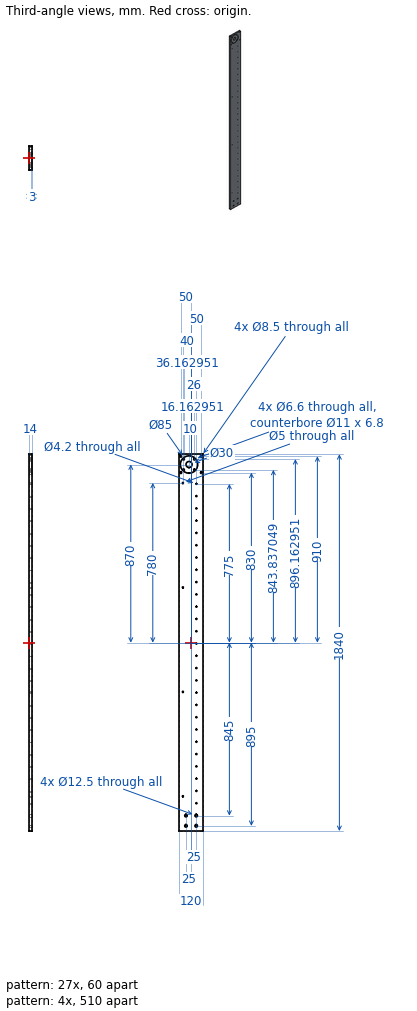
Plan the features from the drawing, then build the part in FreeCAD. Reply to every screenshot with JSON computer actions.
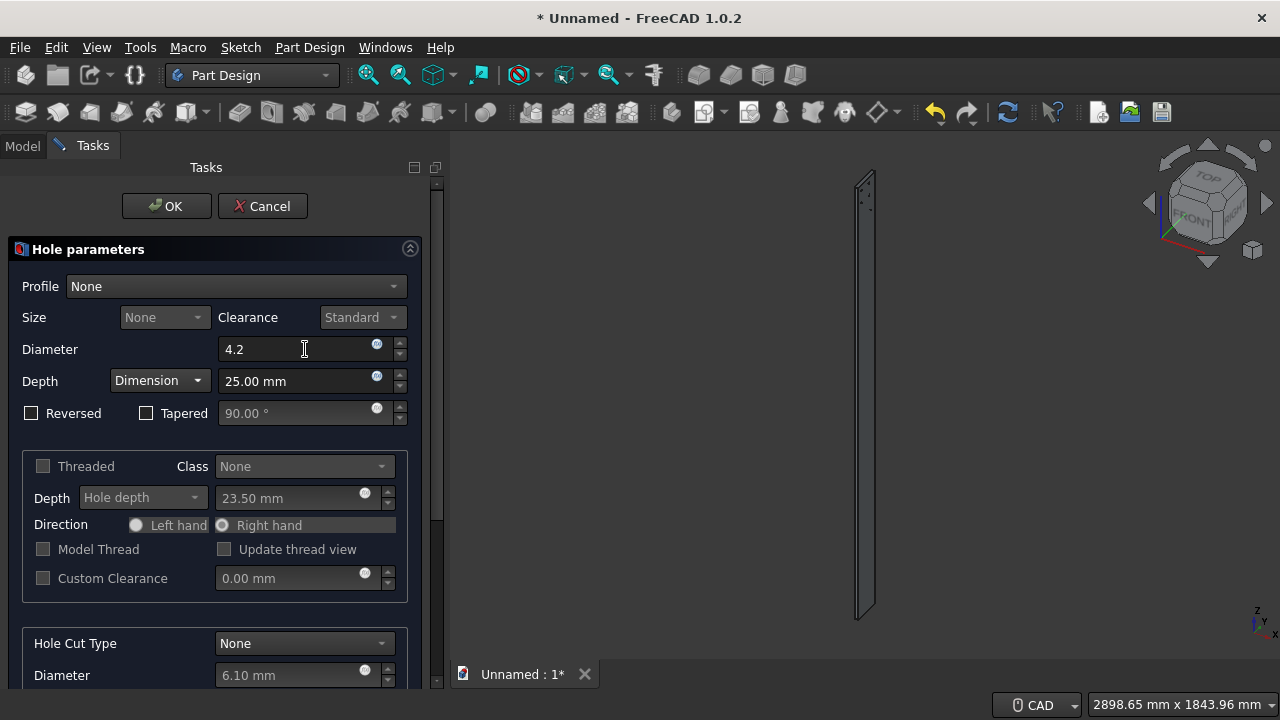
{"action": "left_click", "coordinate": [161, 380]}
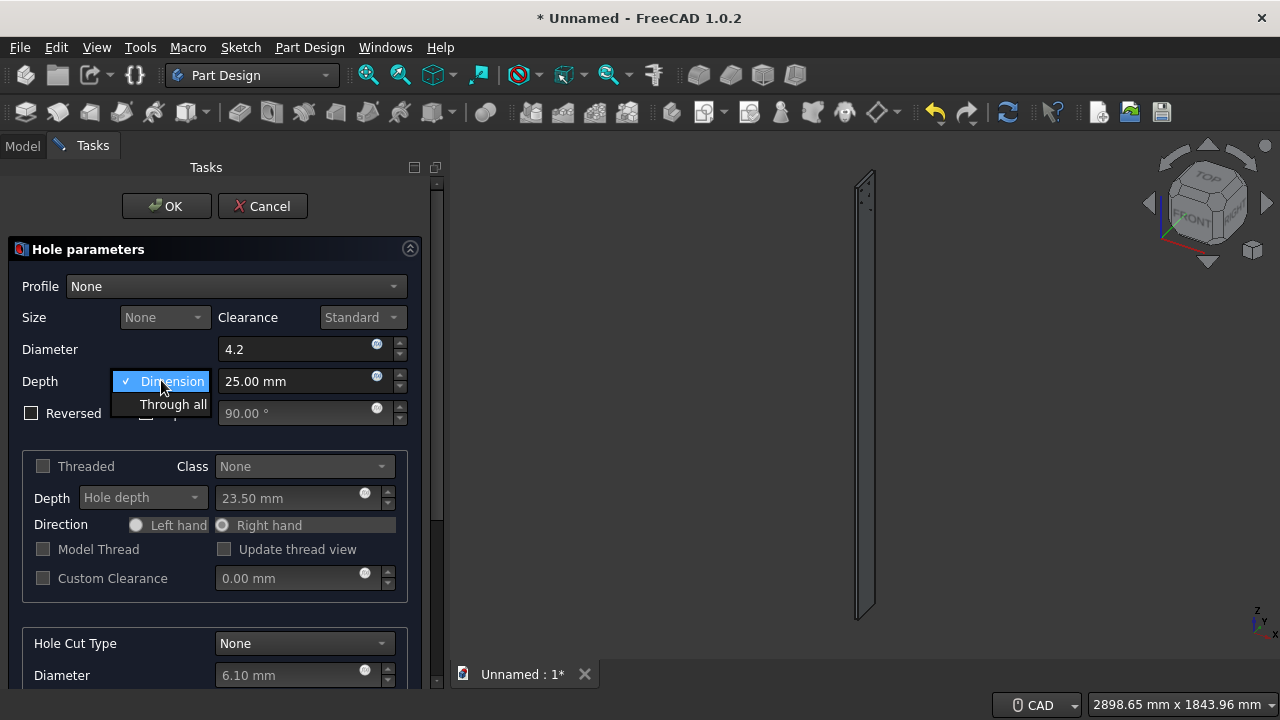
{"action": "left_click", "coordinate": [160, 404]}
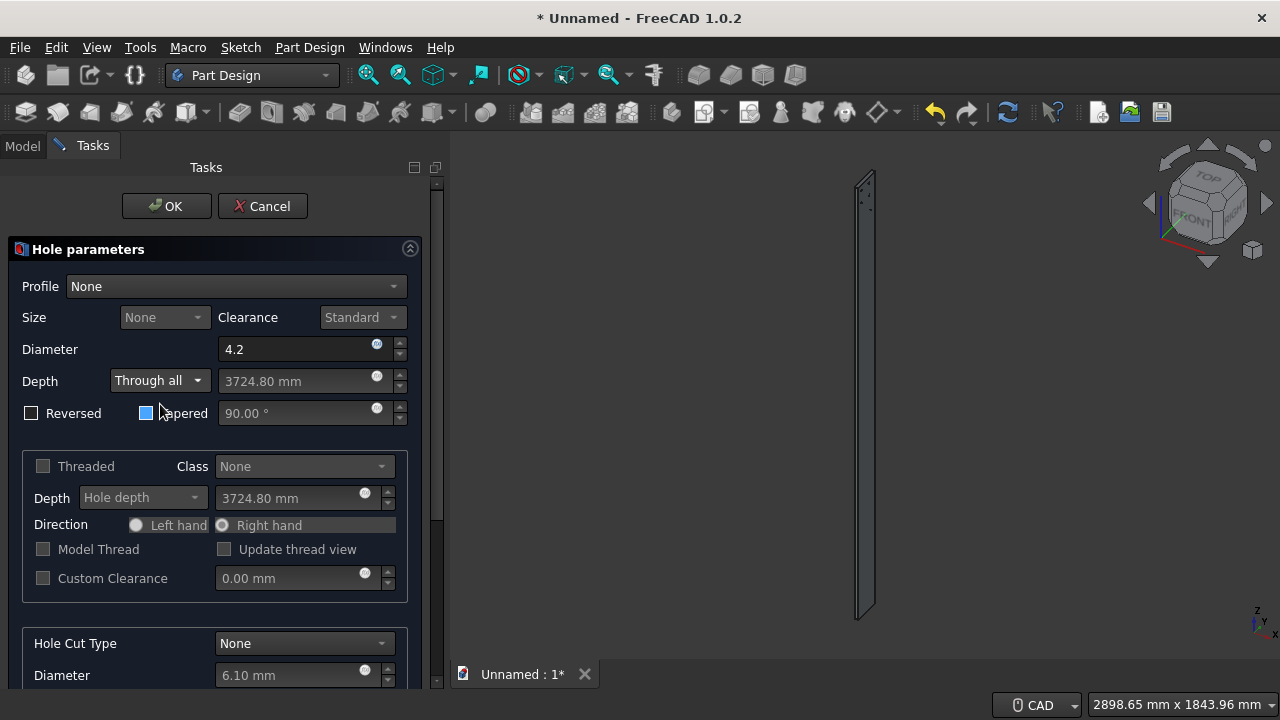
{"action": "left_click", "coordinate": [167, 206]}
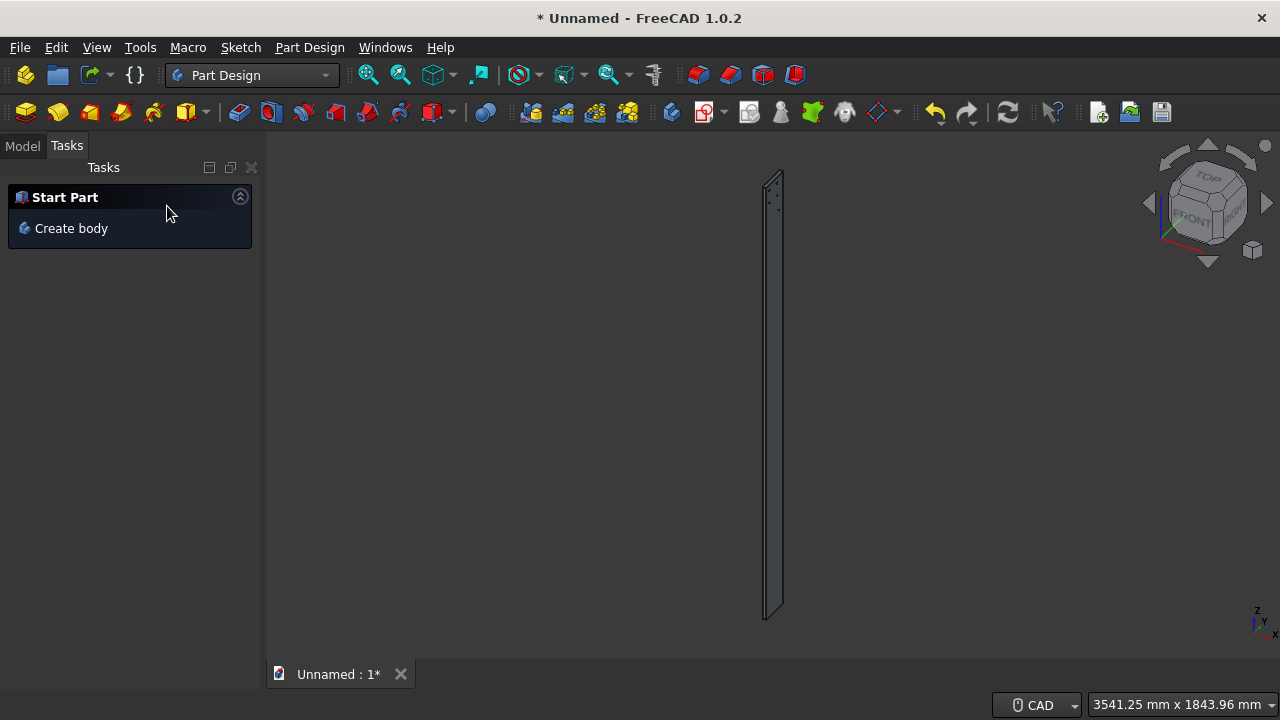
{"action": "left_click", "coordinate": [23, 145]}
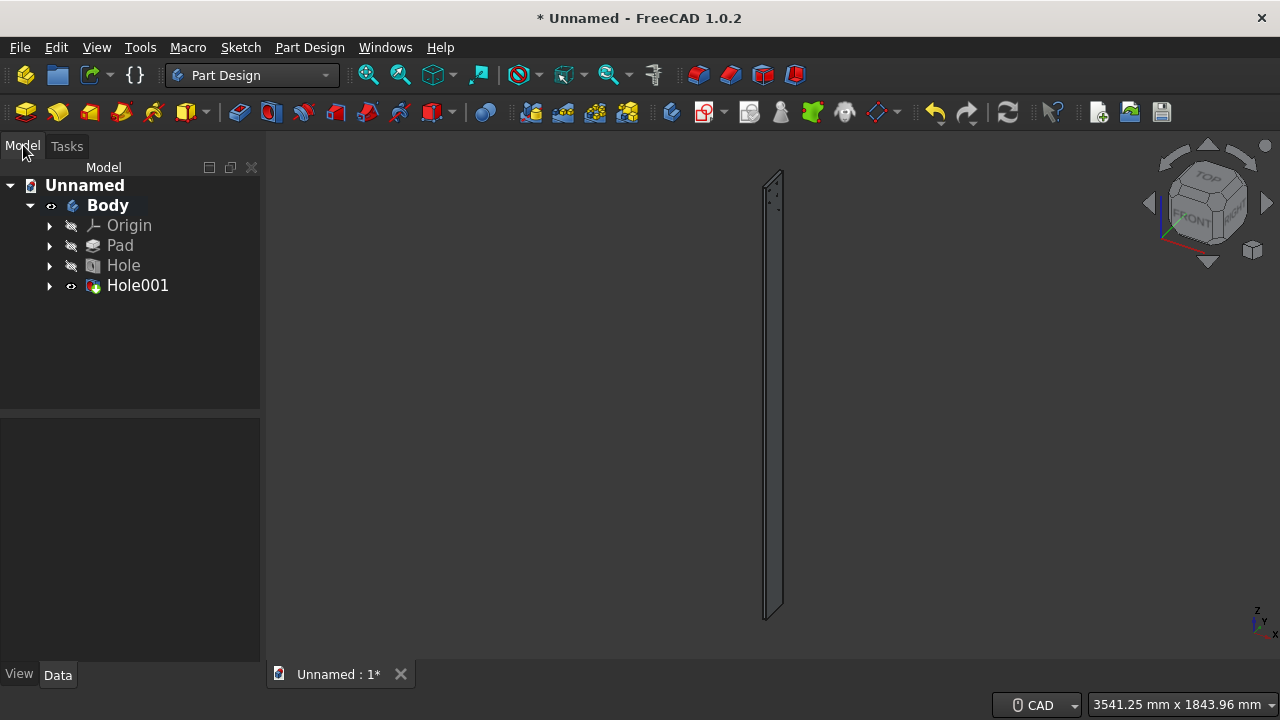
{"action": "left_click", "coordinate": [116, 286]}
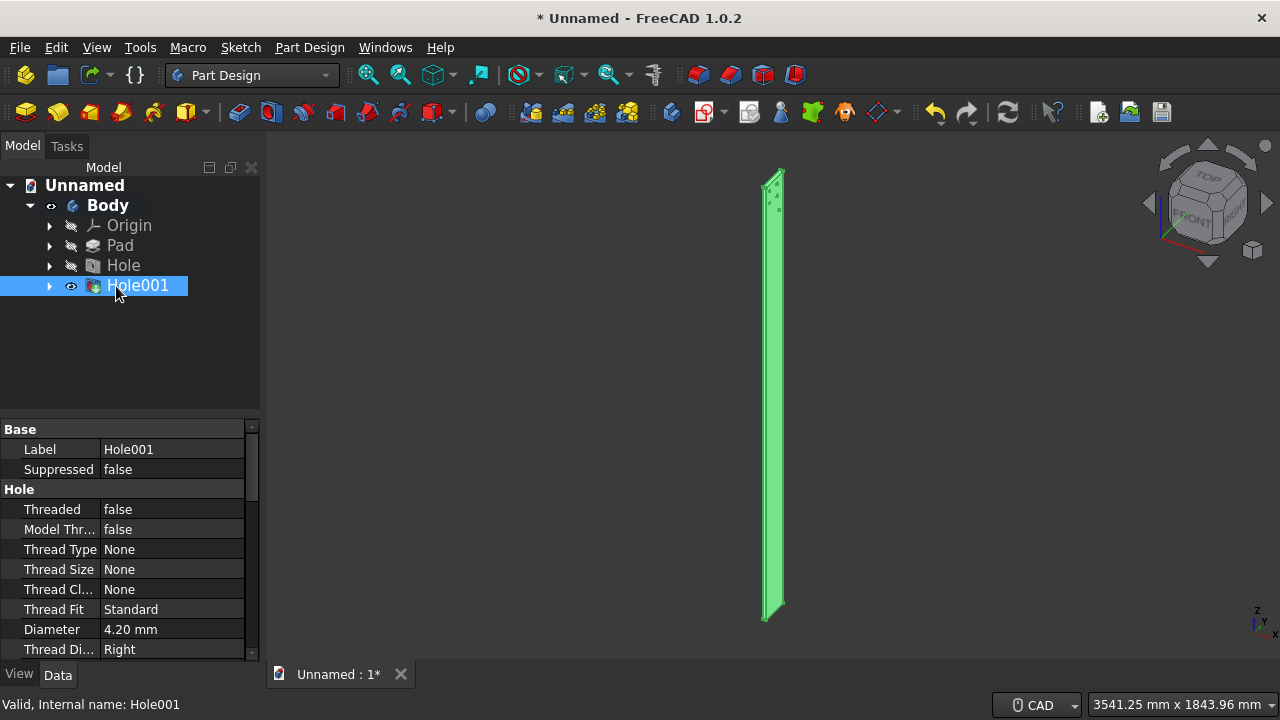
{"action": "left_click", "coordinate": [564, 112]}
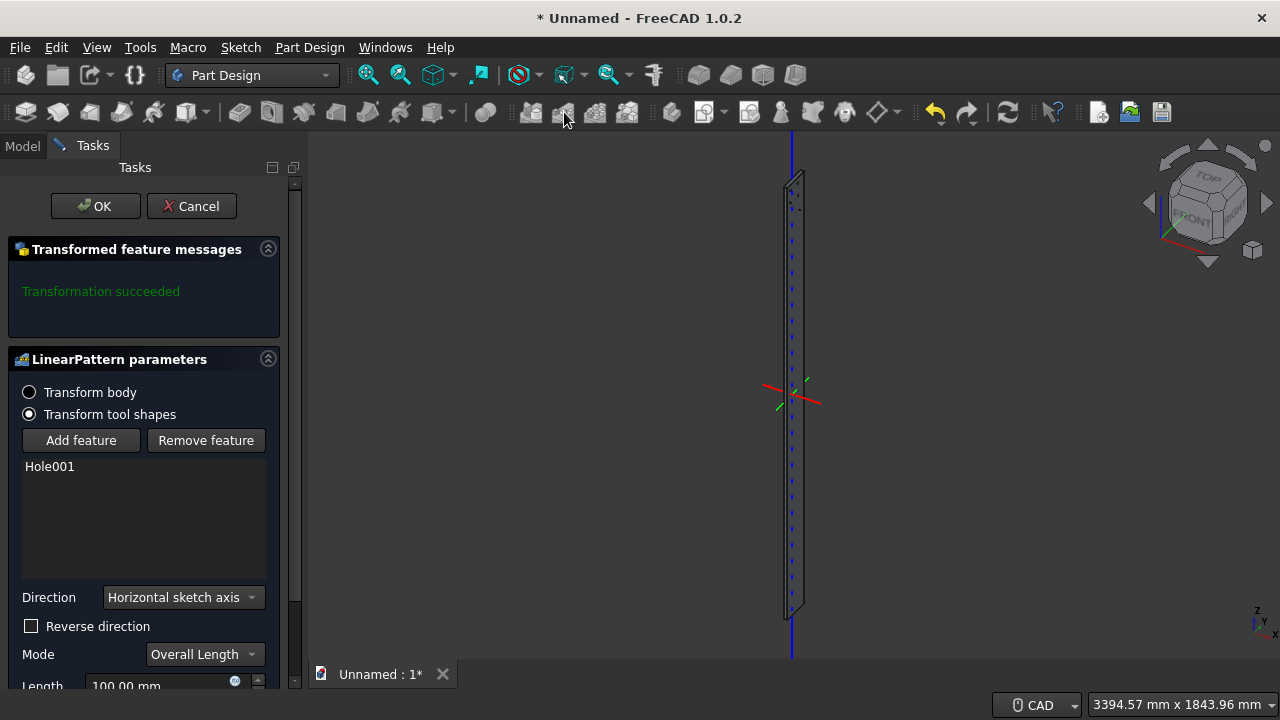
{"action": "left_click", "coordinate": [184, 598]}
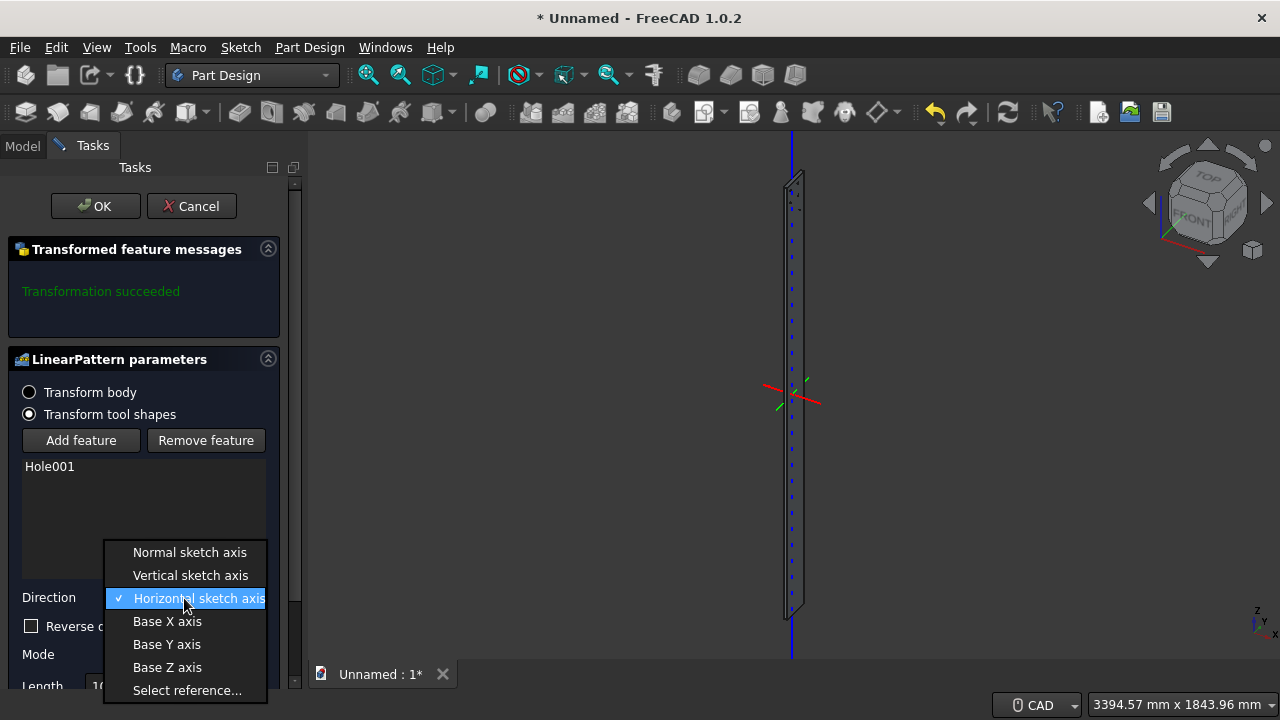
{"action": "left_click", "coordinate": [184, 668]}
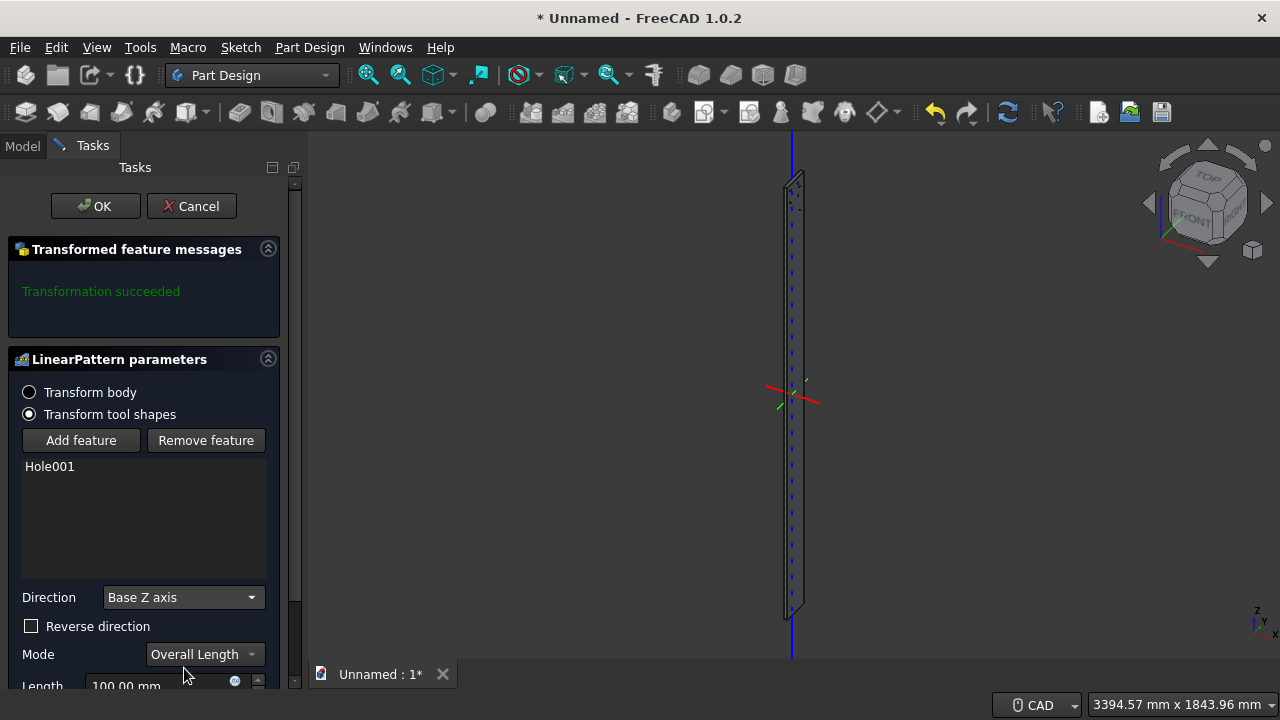
{"action": "left_click", "coordinate": [206, 654]}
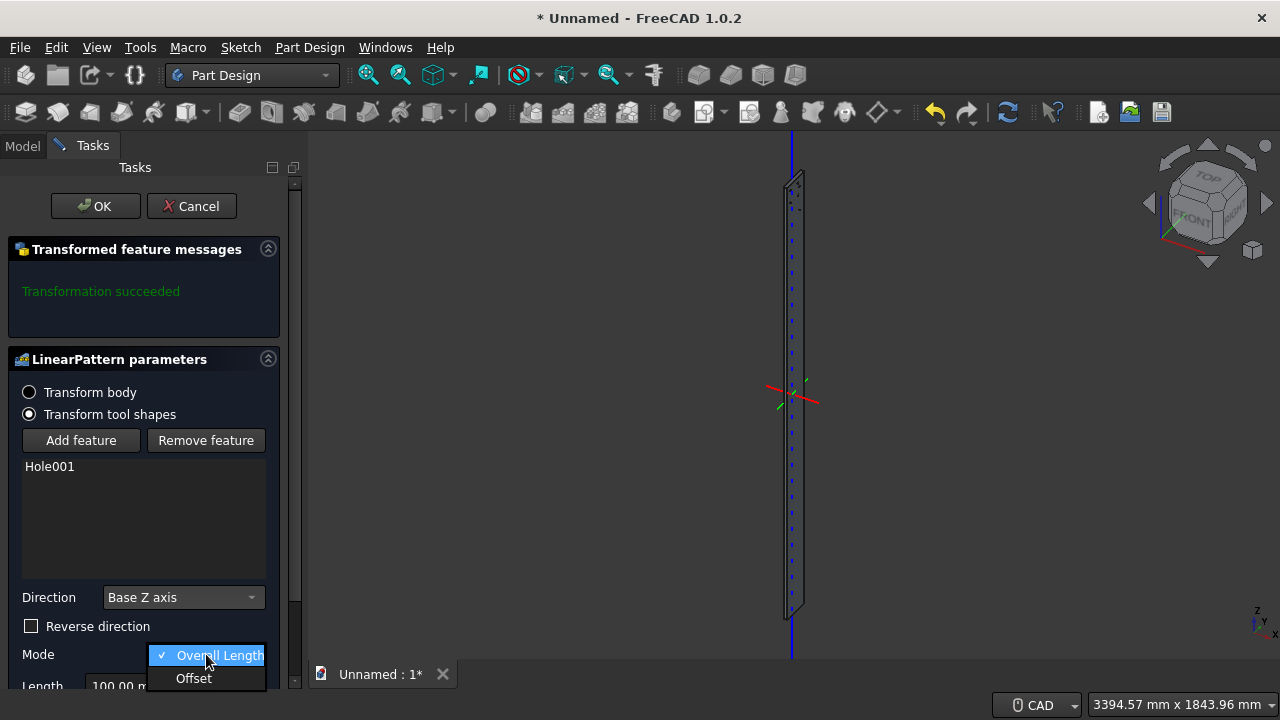
{"action": "left_click", "coordinate": [206, 678]}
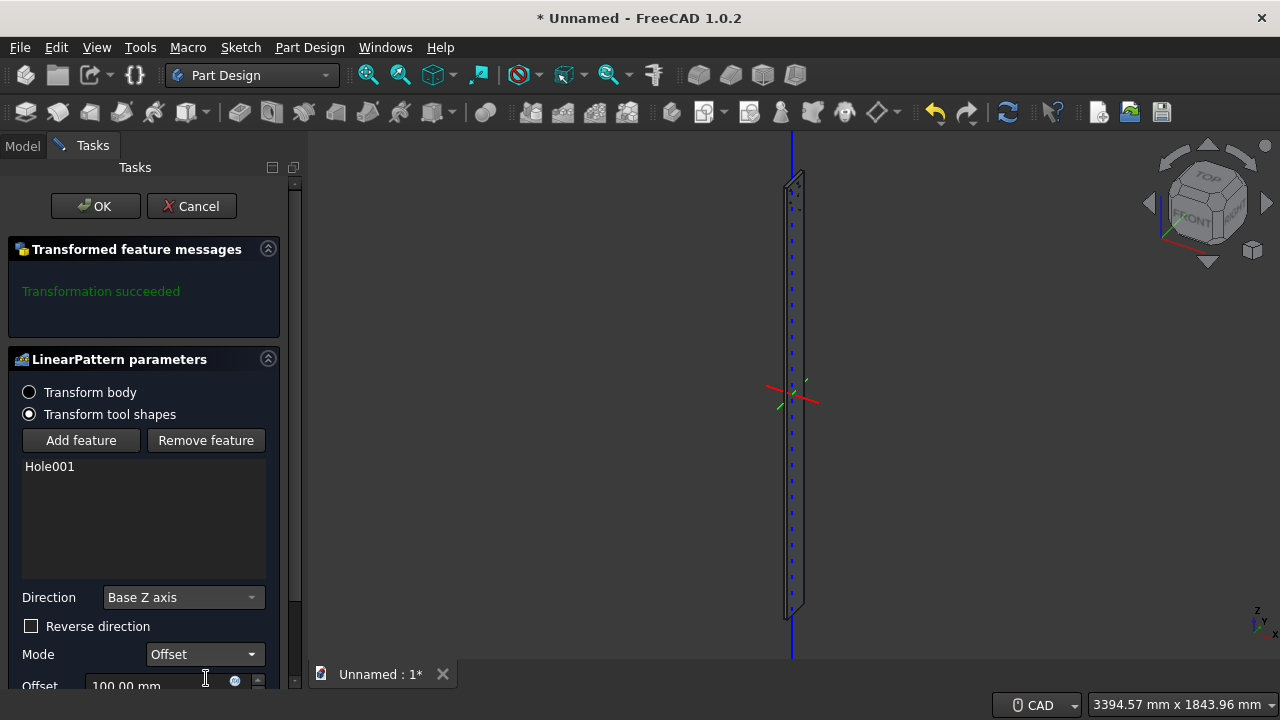
{"action": "scroll", "coordinate": [295, 432], "scroll_direction": "down", "scroll_amount": 2}